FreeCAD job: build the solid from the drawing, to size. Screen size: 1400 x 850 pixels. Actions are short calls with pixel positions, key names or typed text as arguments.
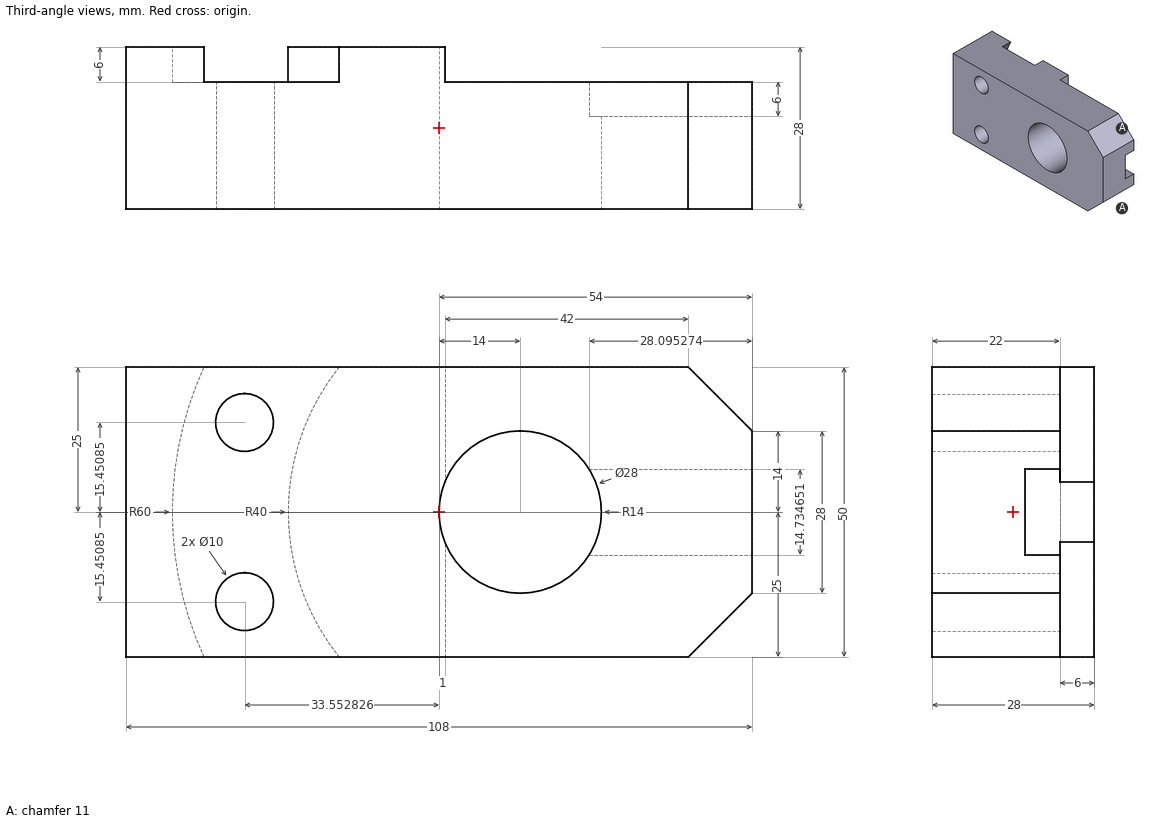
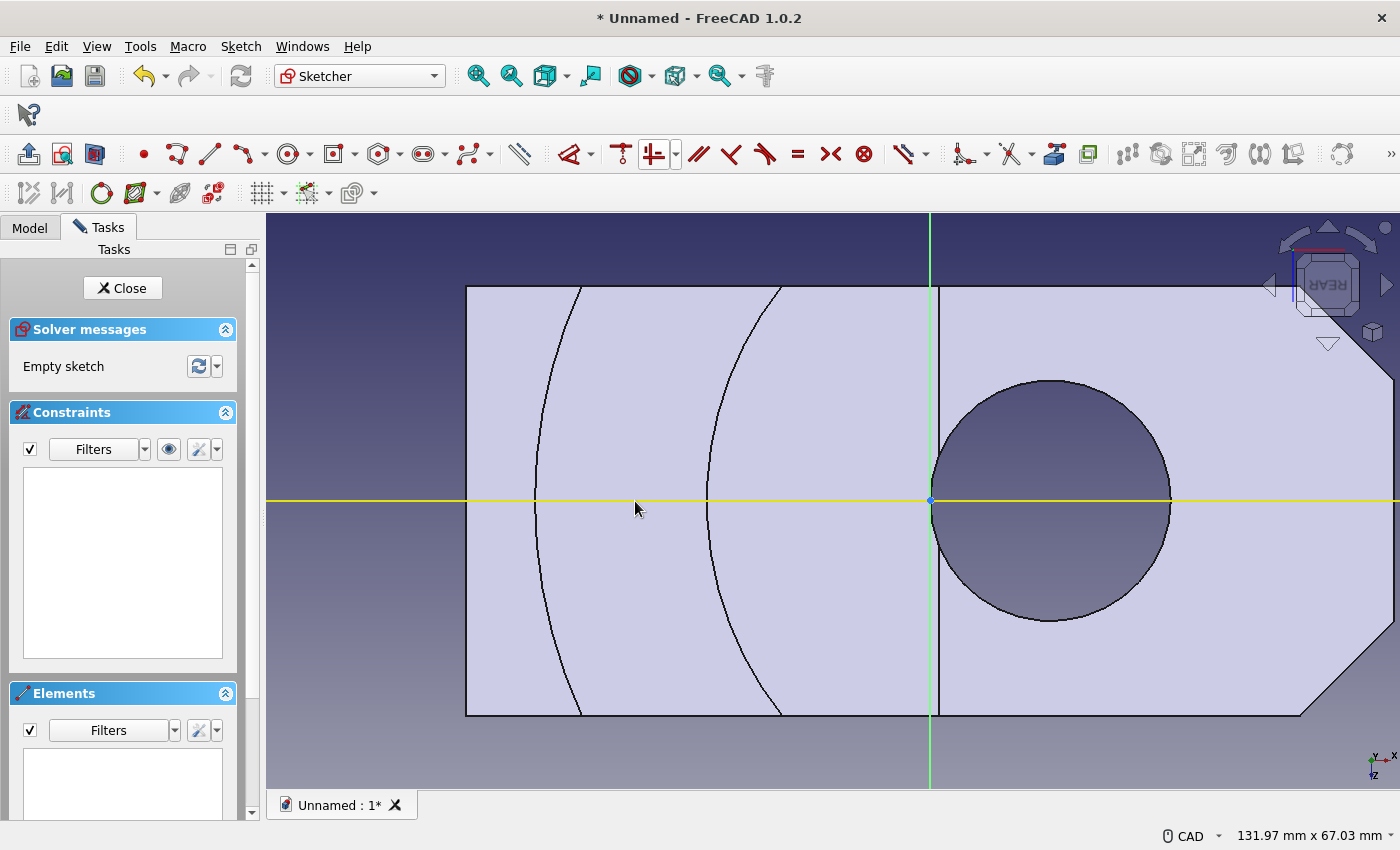
click(288, 154)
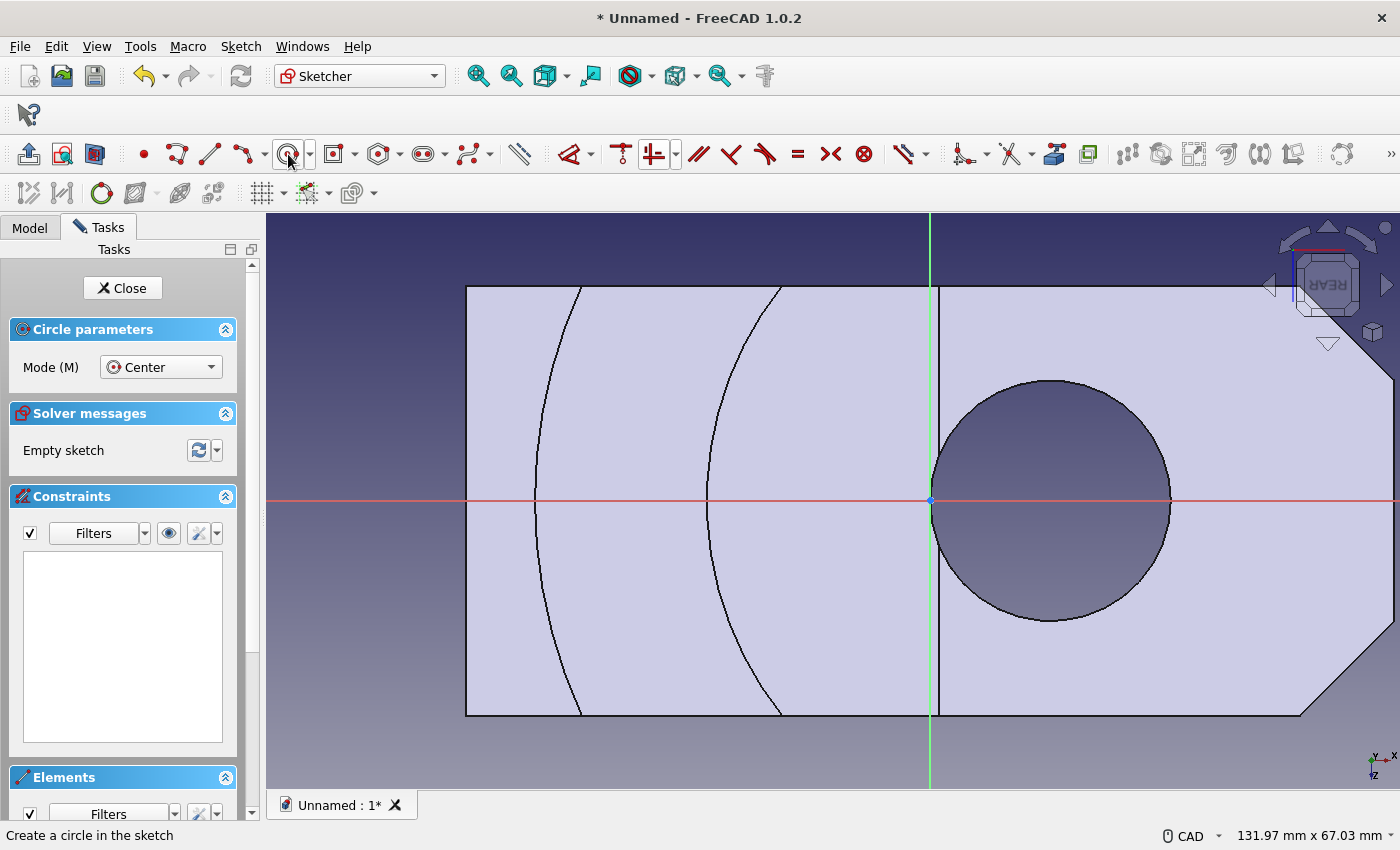
click(642, 368)
move(672, 338)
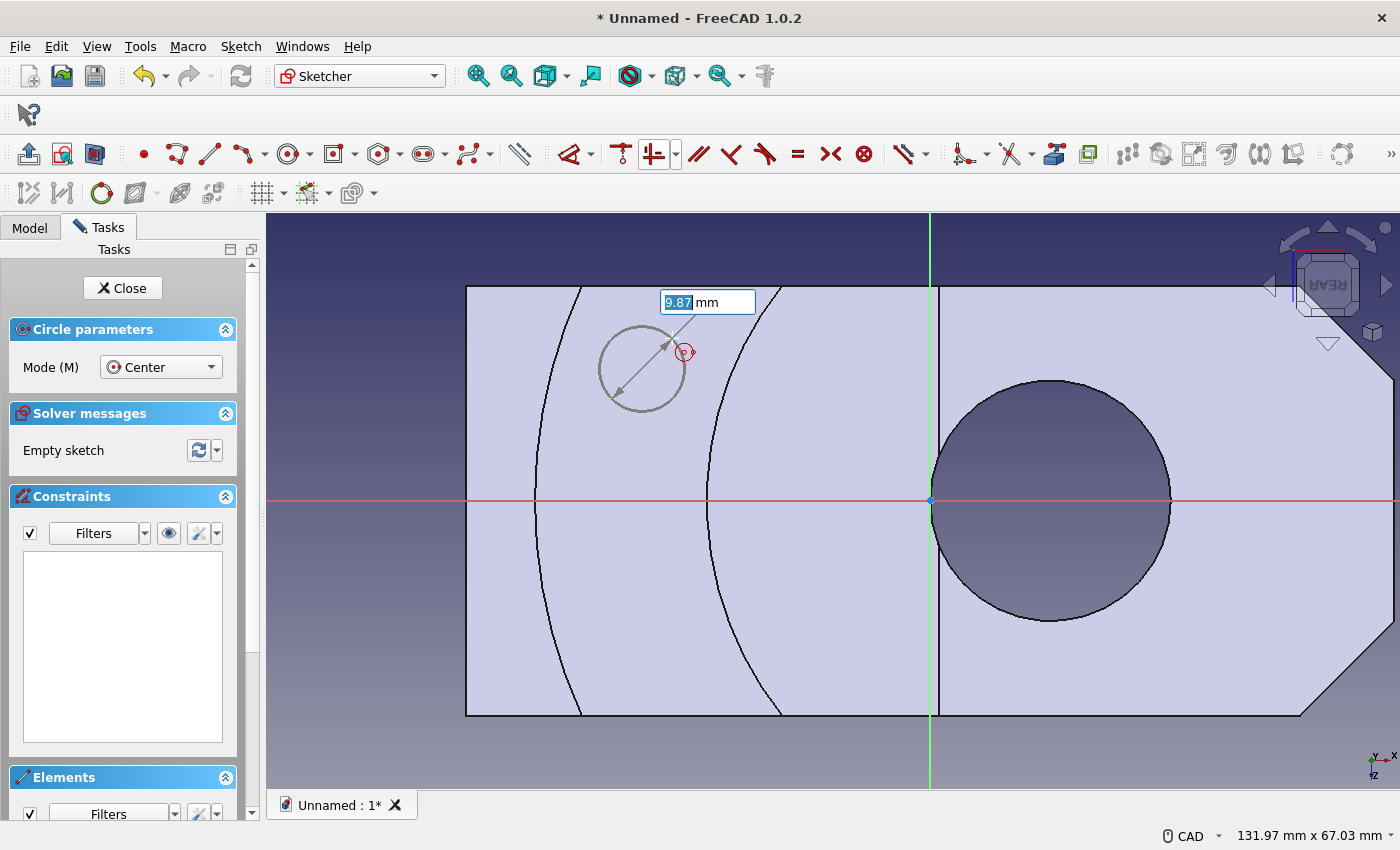
text(10)
key(Return)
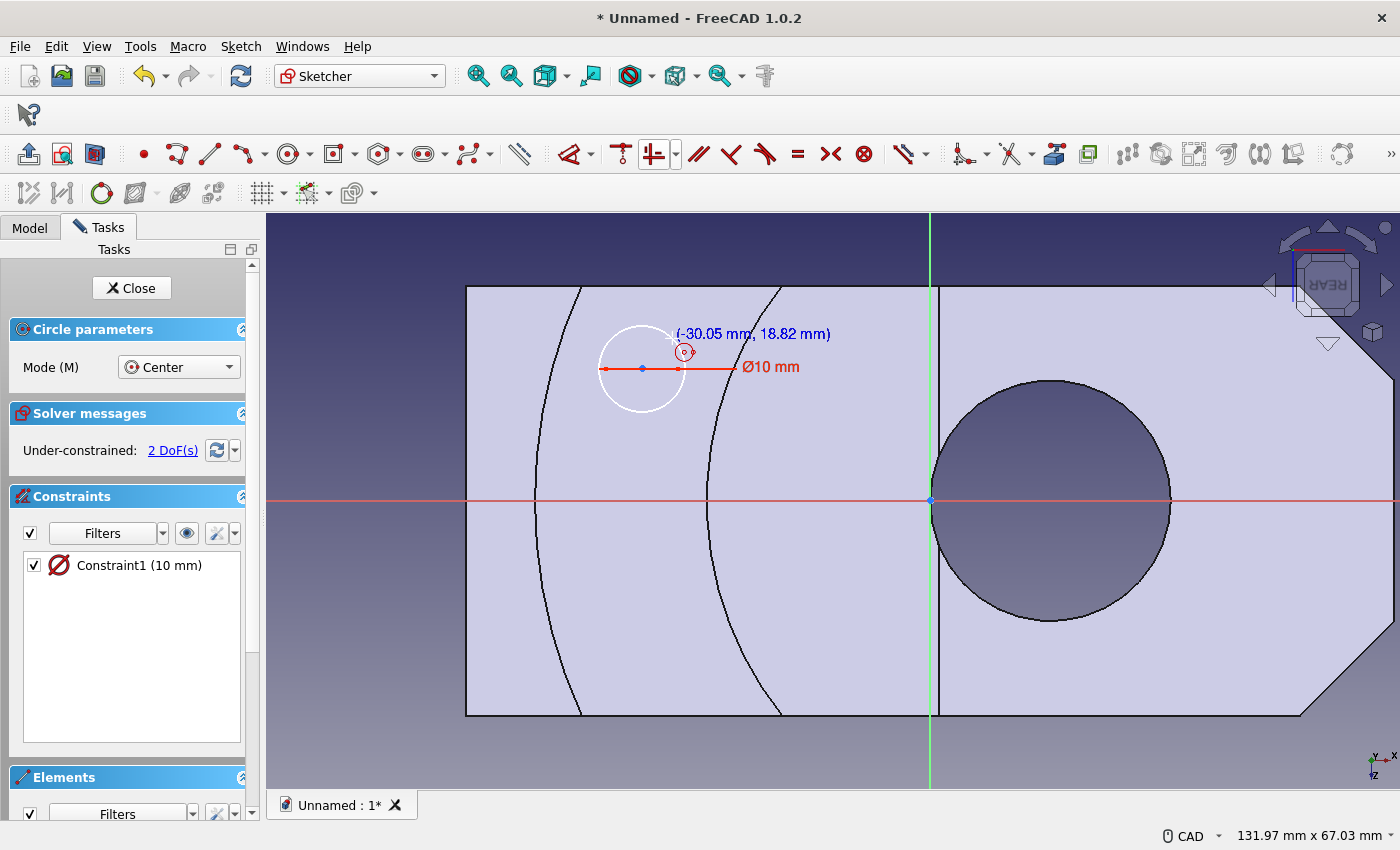
click(642, 634)
move(672, 603)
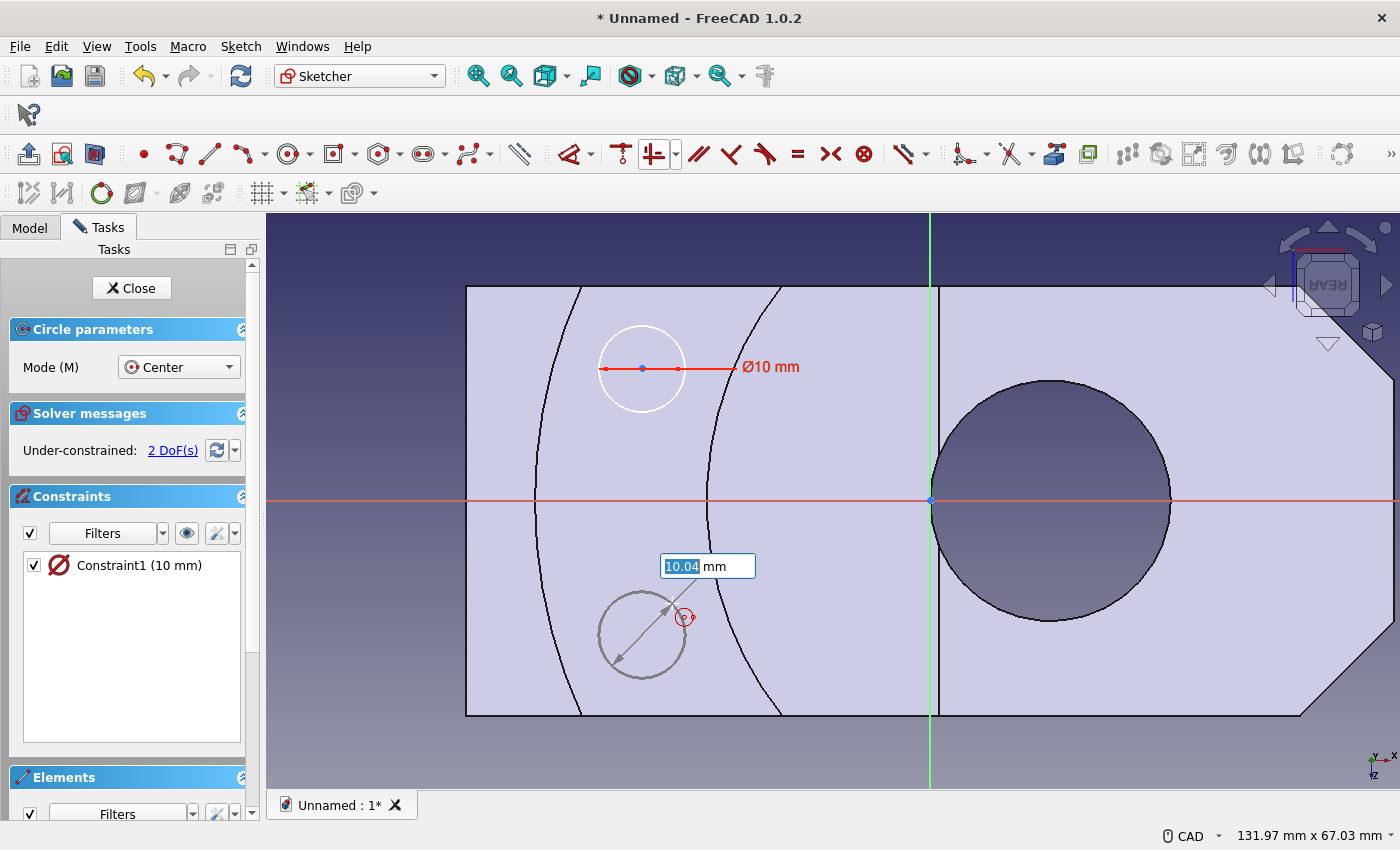
text(10)
key(Return)
key(Escape)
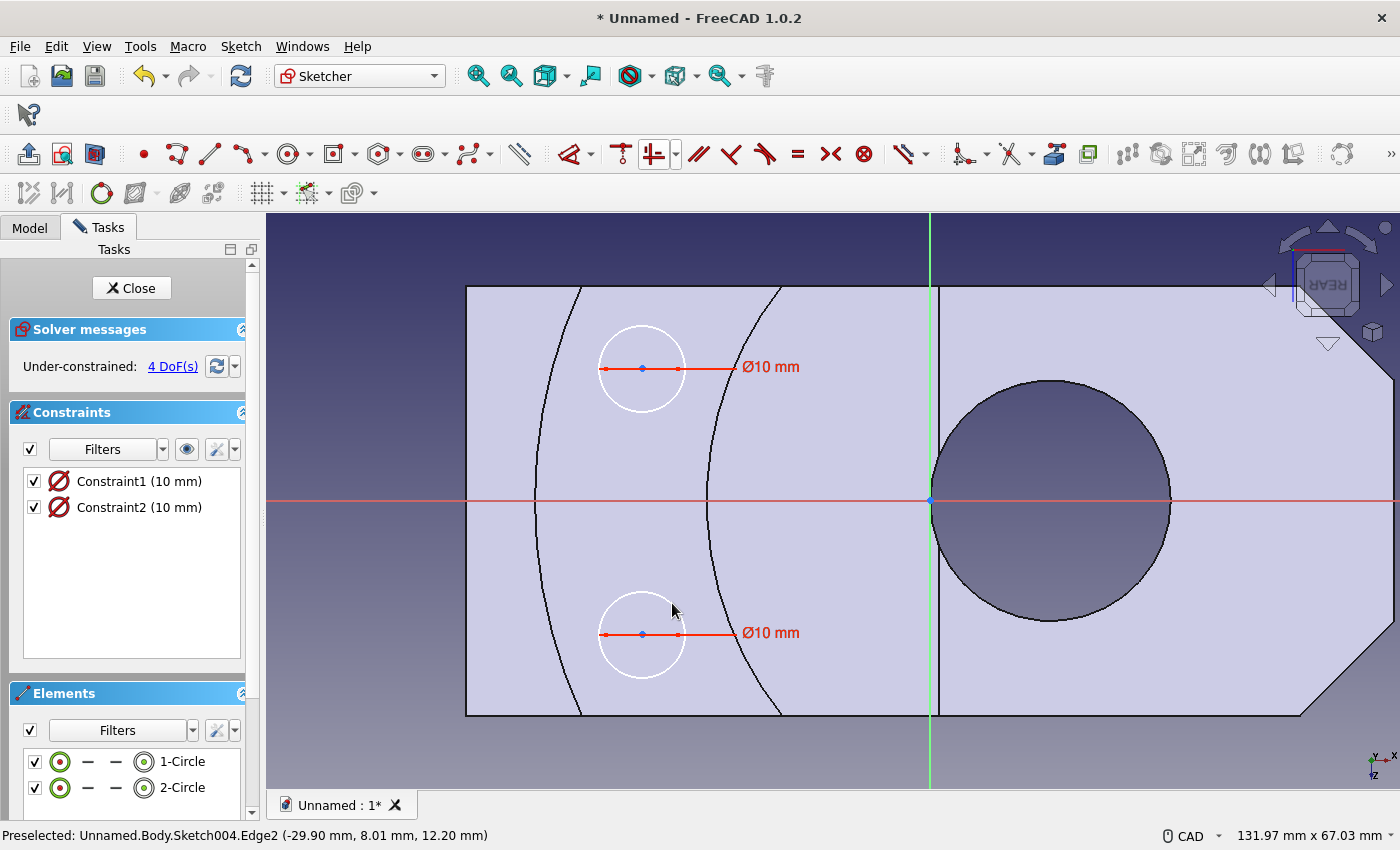
click(642, 369)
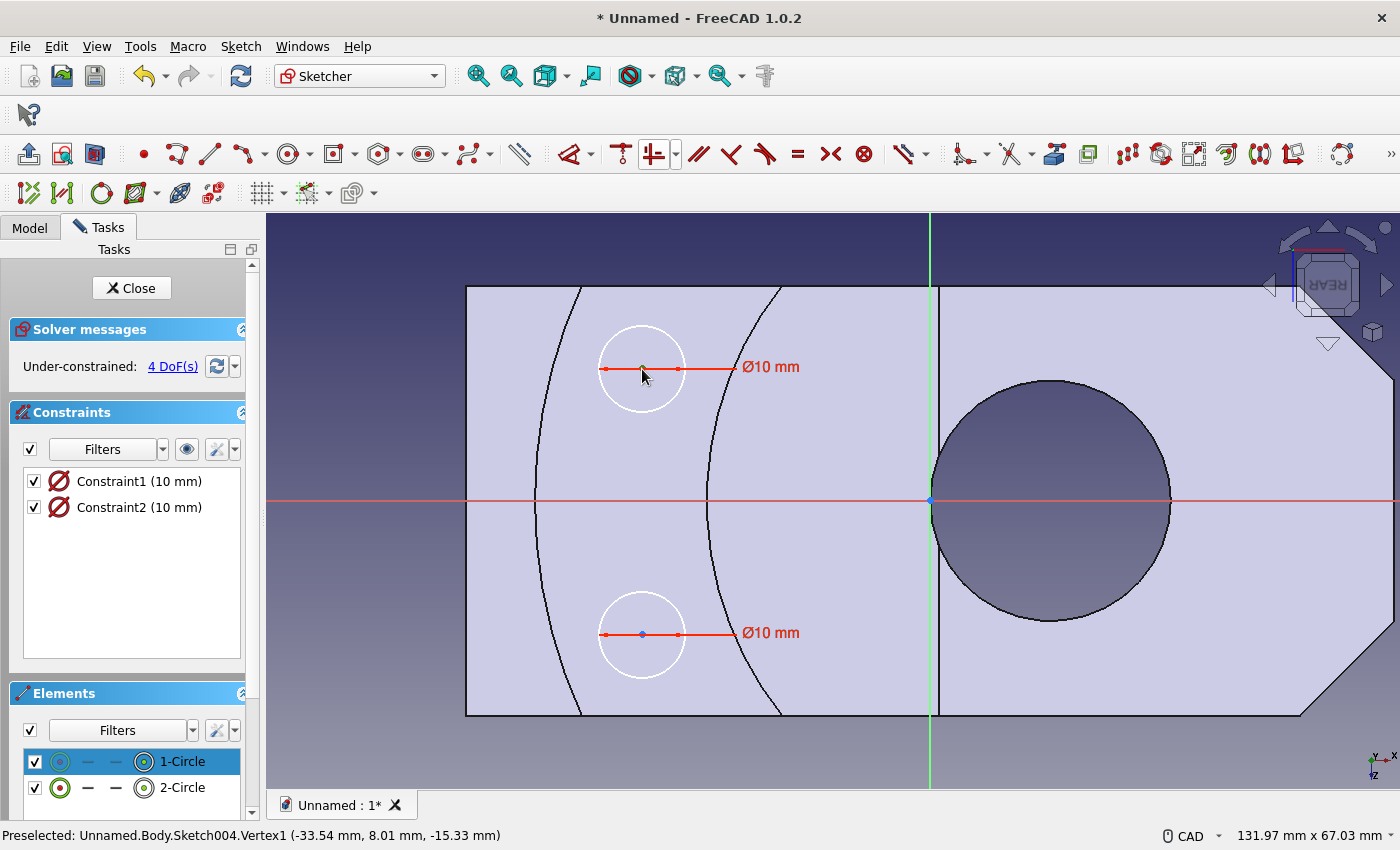
click(642, 635)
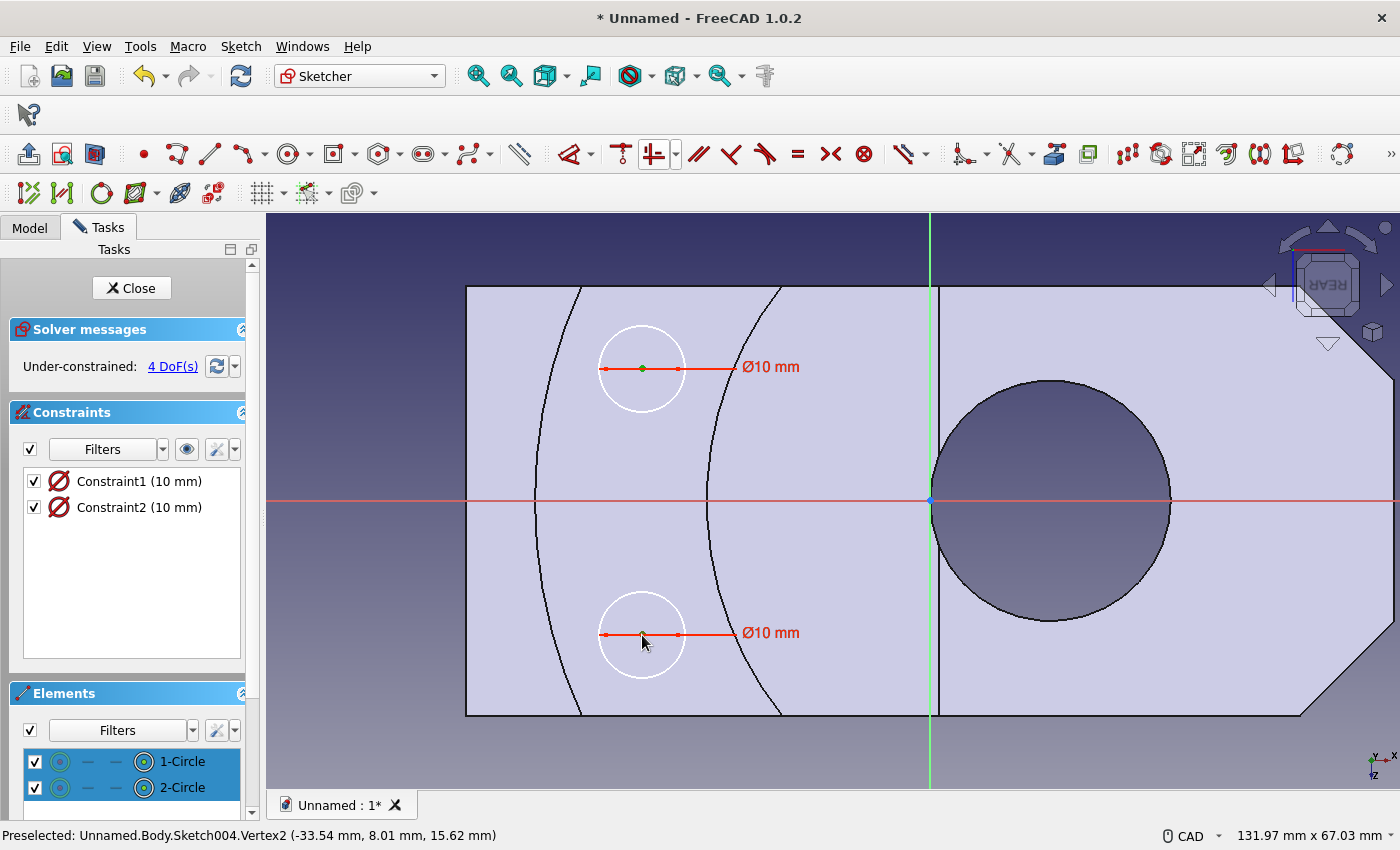
key(v)